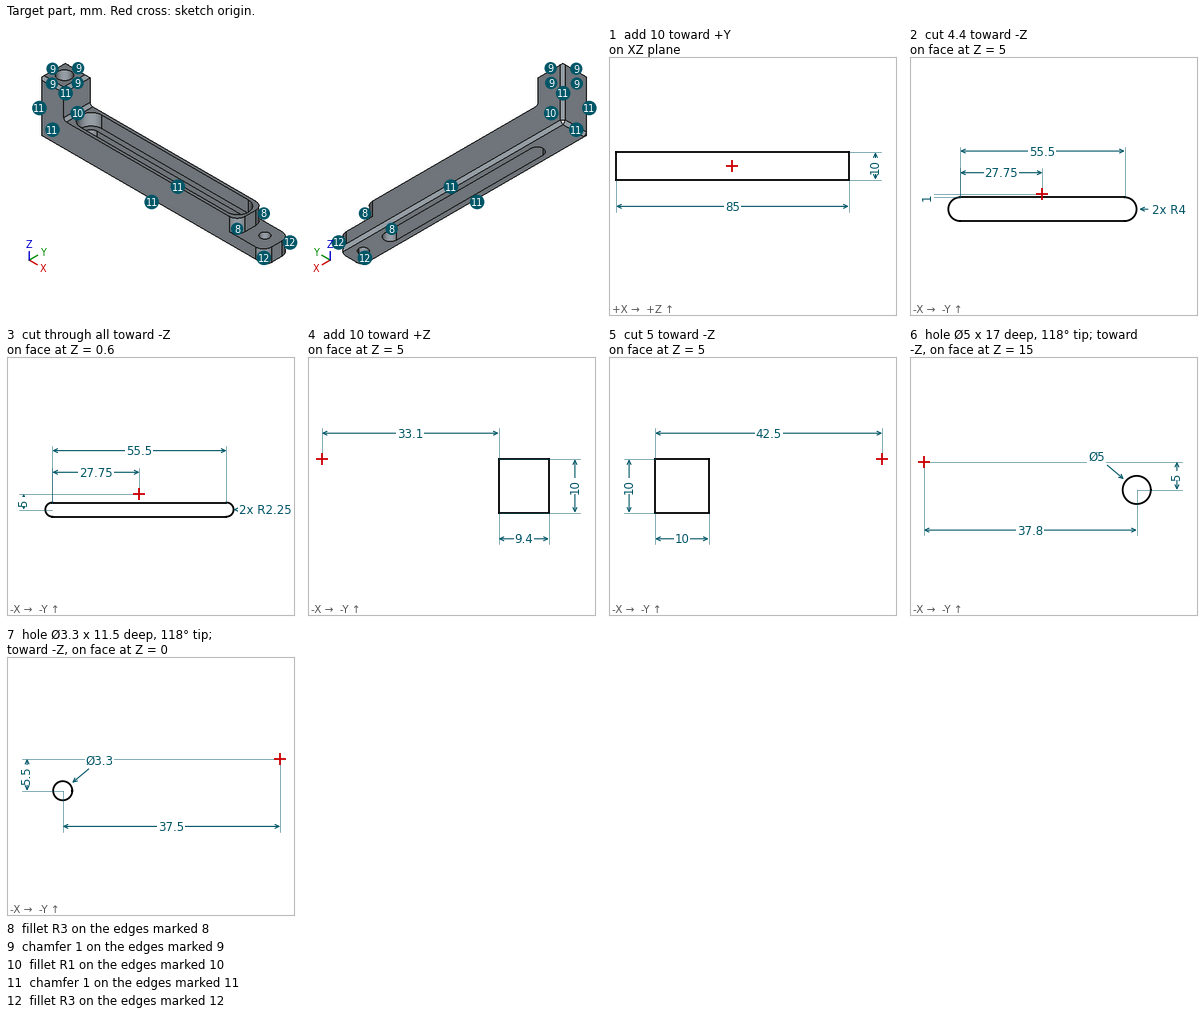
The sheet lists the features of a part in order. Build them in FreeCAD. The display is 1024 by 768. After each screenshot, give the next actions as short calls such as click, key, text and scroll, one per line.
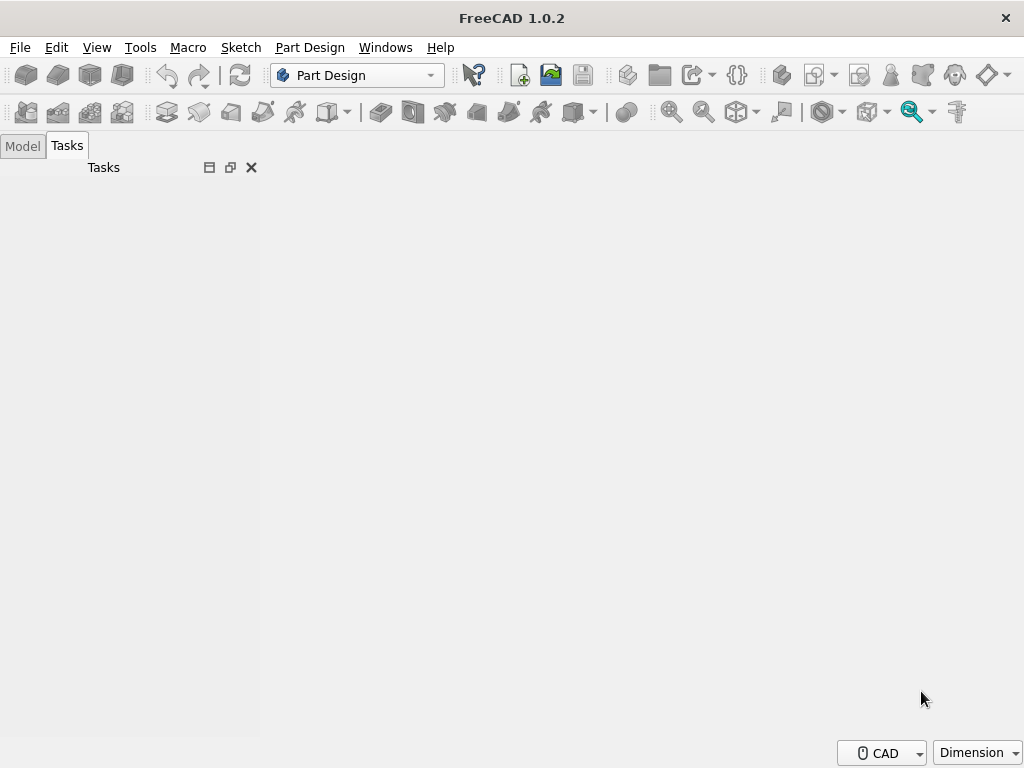
key(ctrl+n)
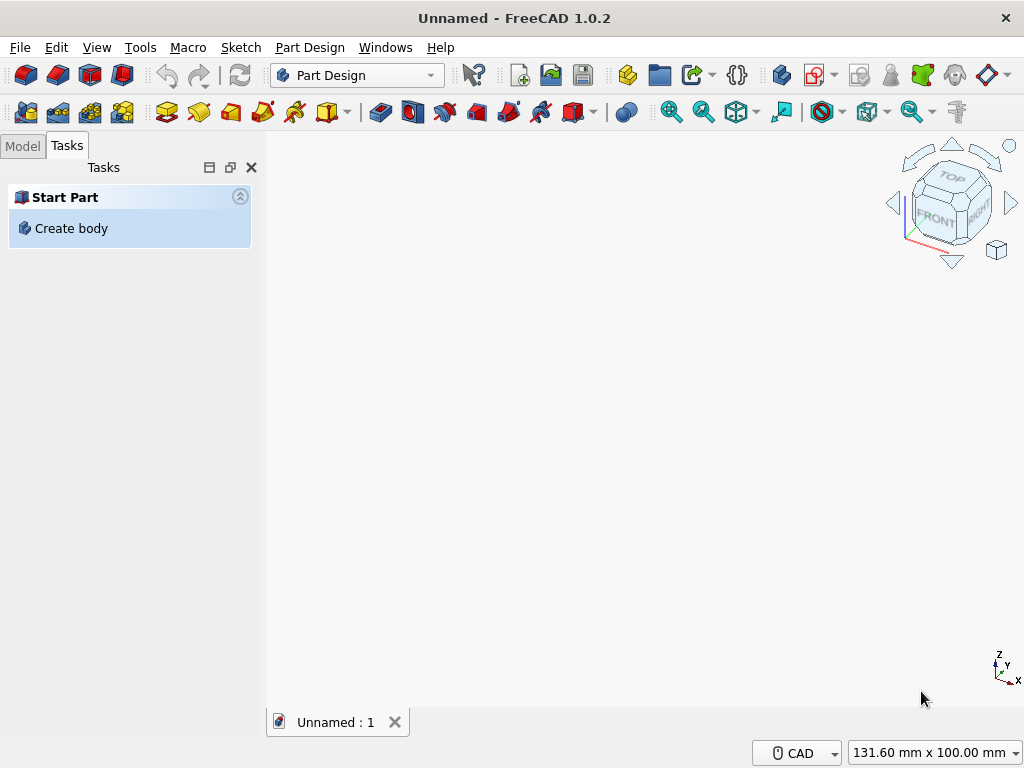
click(814, 76)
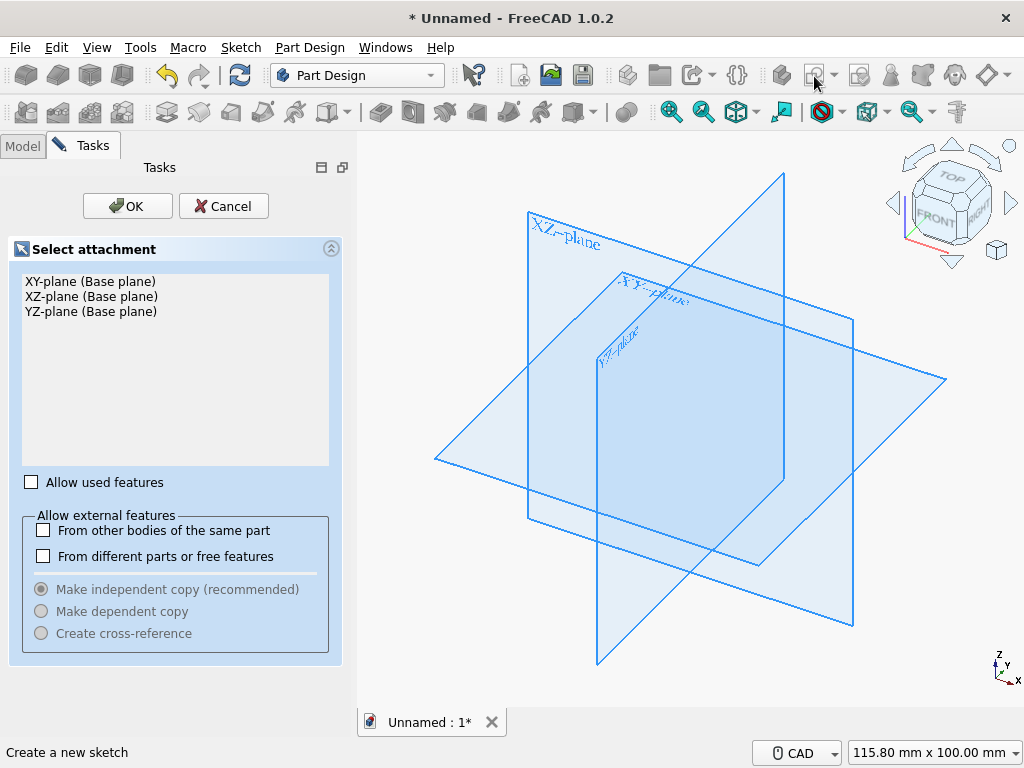
click(82, 296)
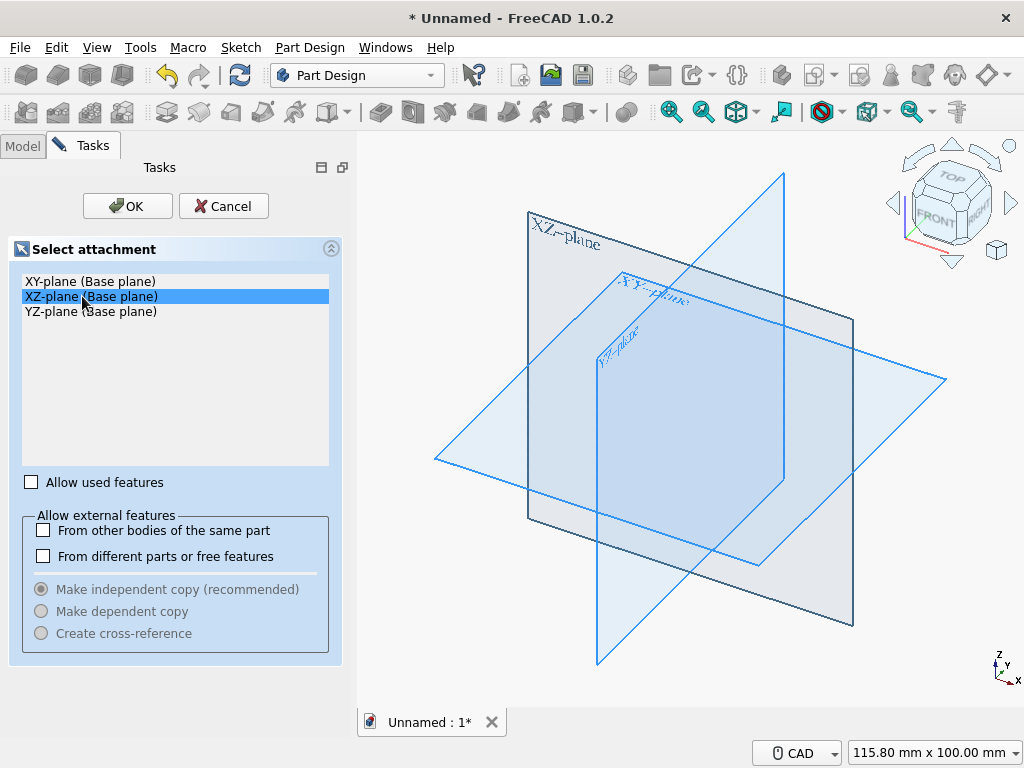
click(128, 206)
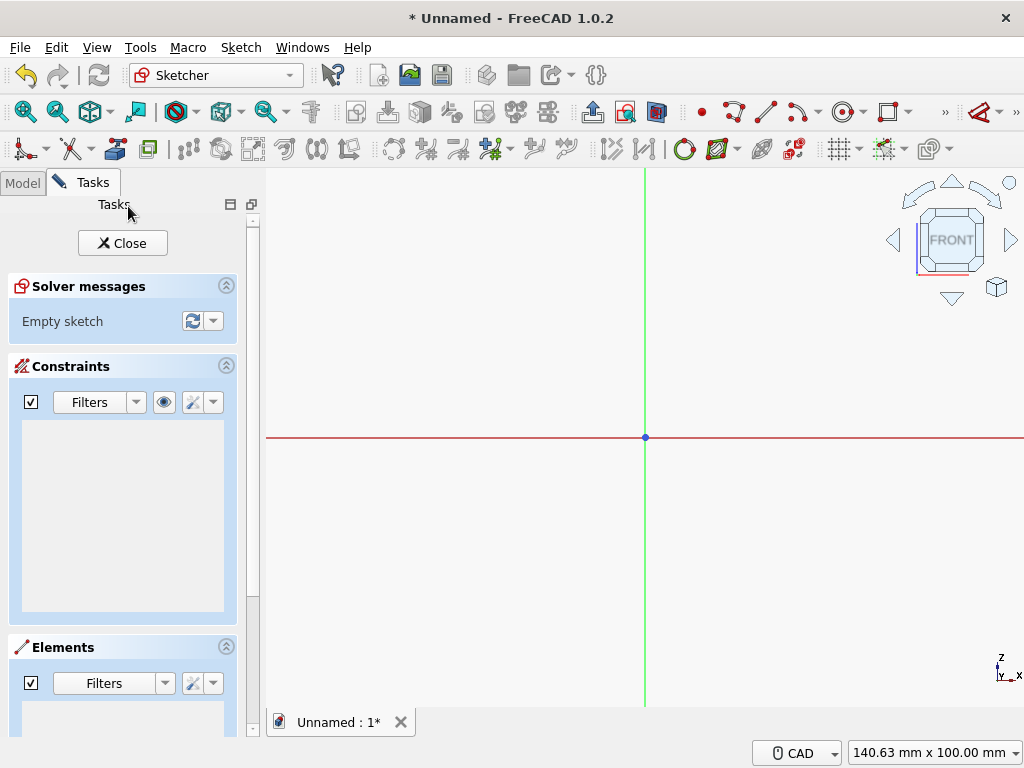
scroll(294, 437, down, 1)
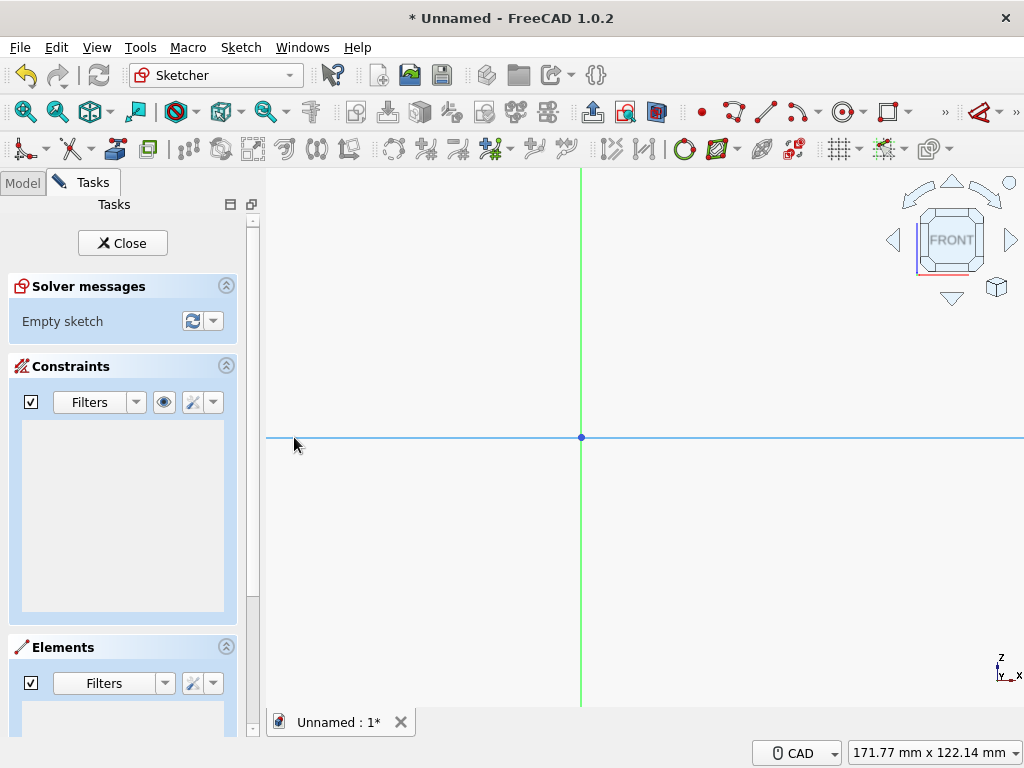
key(g)
key(v)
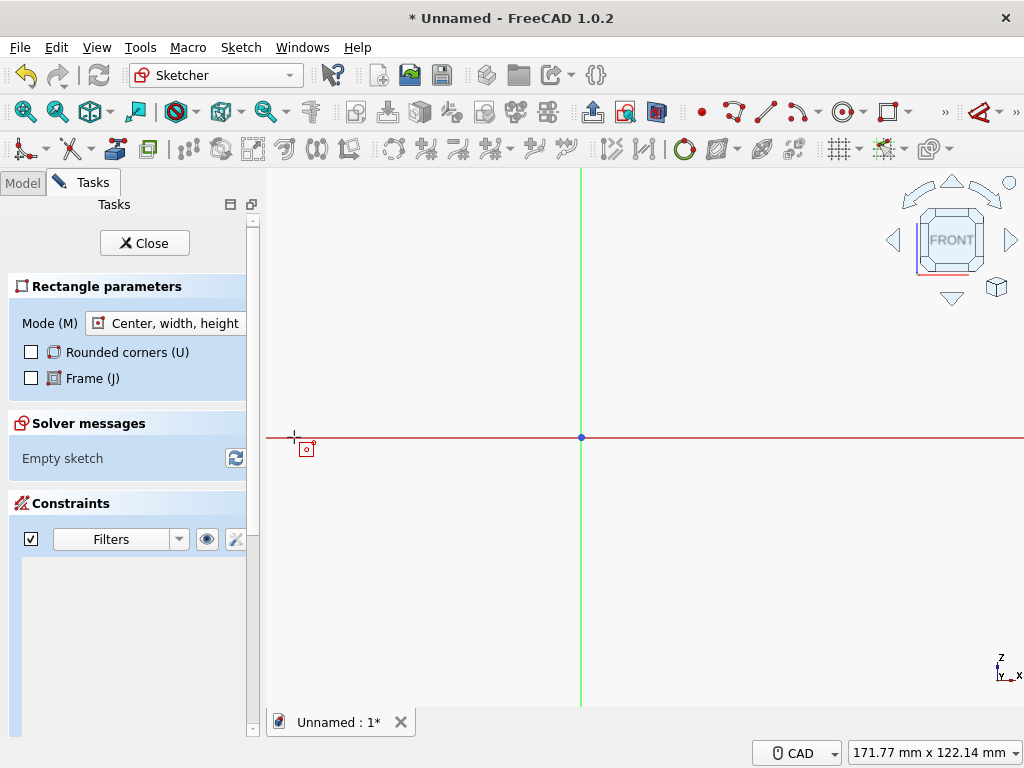
click(581, 438)
click(769, 415)
key(Escape)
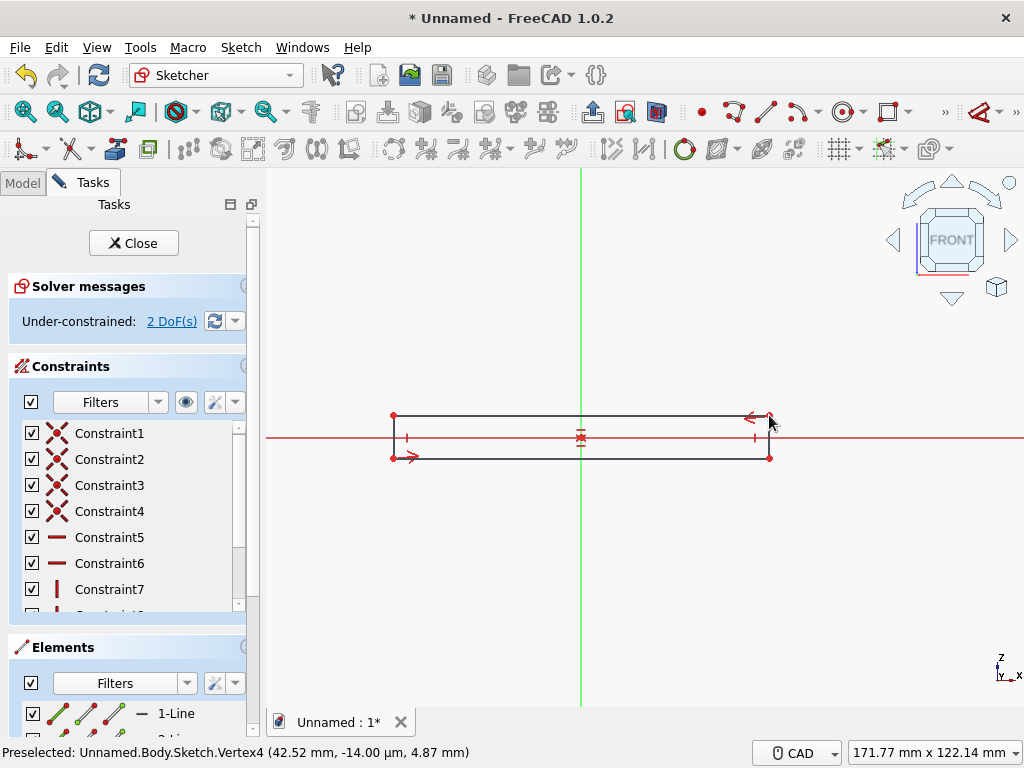
click(980, 112)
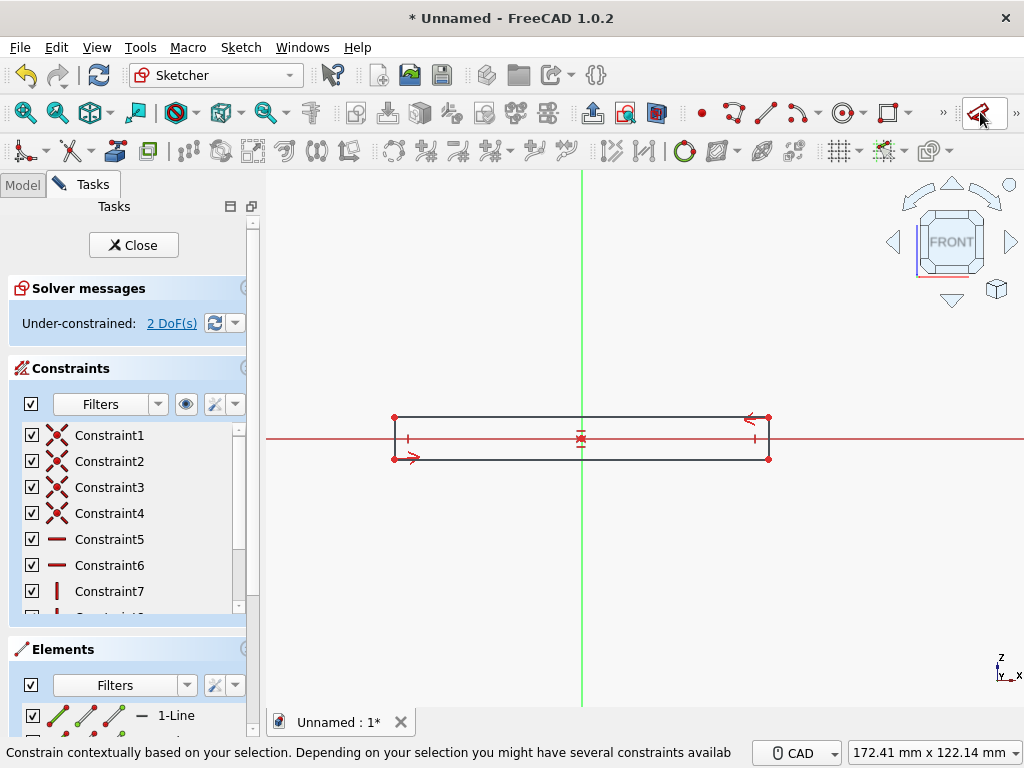
click(507, 460)
click(496, 494)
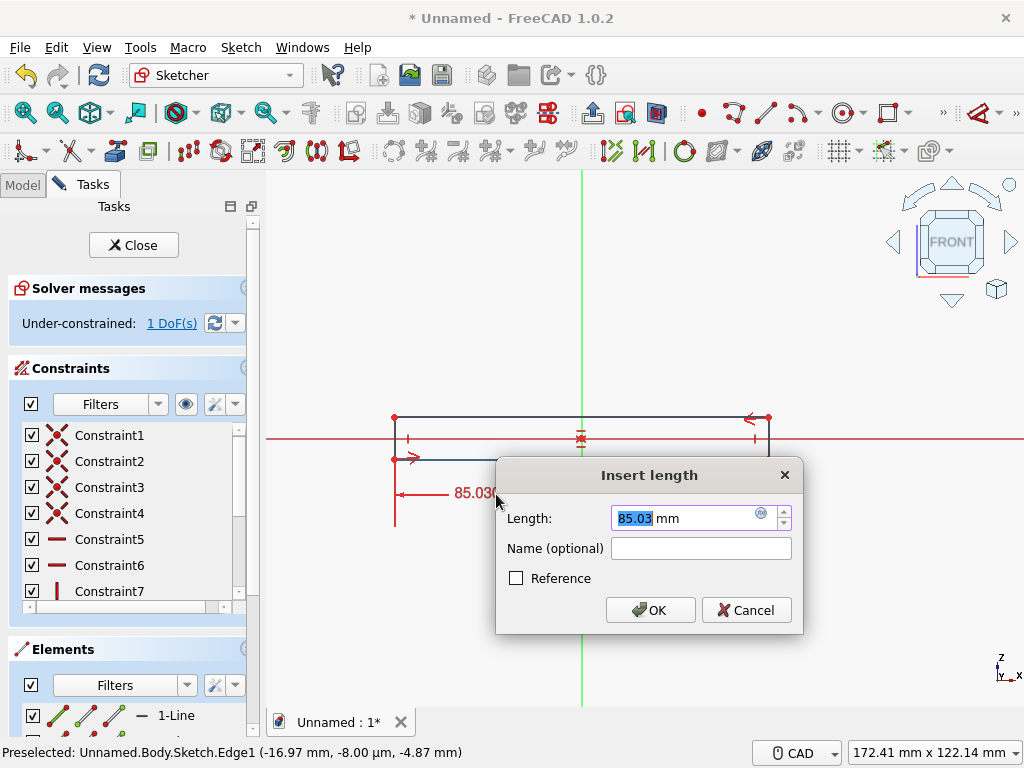
text(85)
key(Return)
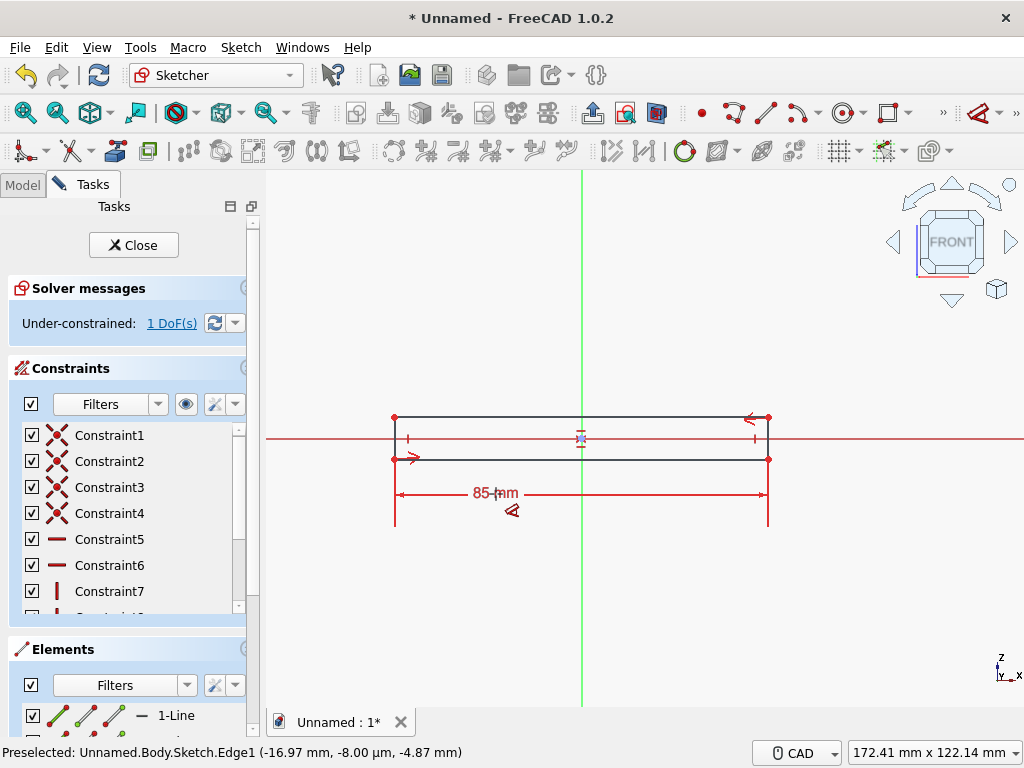
click(768, 438)
click(802, 424)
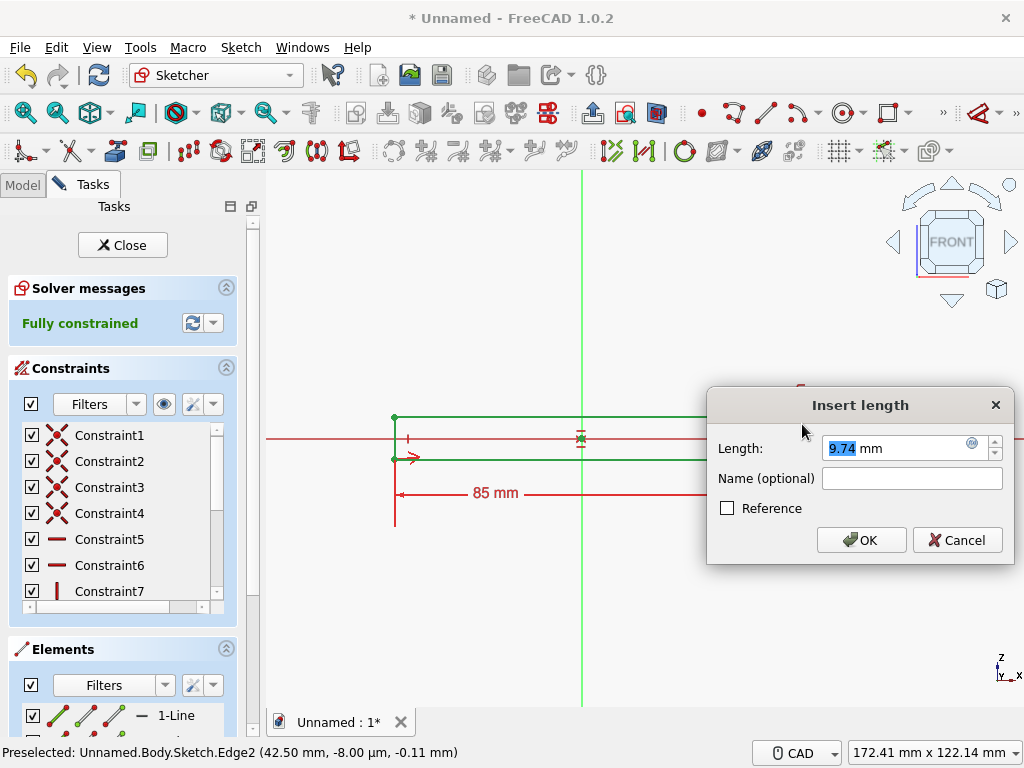
text(10)
key(Return)
key(Escape)